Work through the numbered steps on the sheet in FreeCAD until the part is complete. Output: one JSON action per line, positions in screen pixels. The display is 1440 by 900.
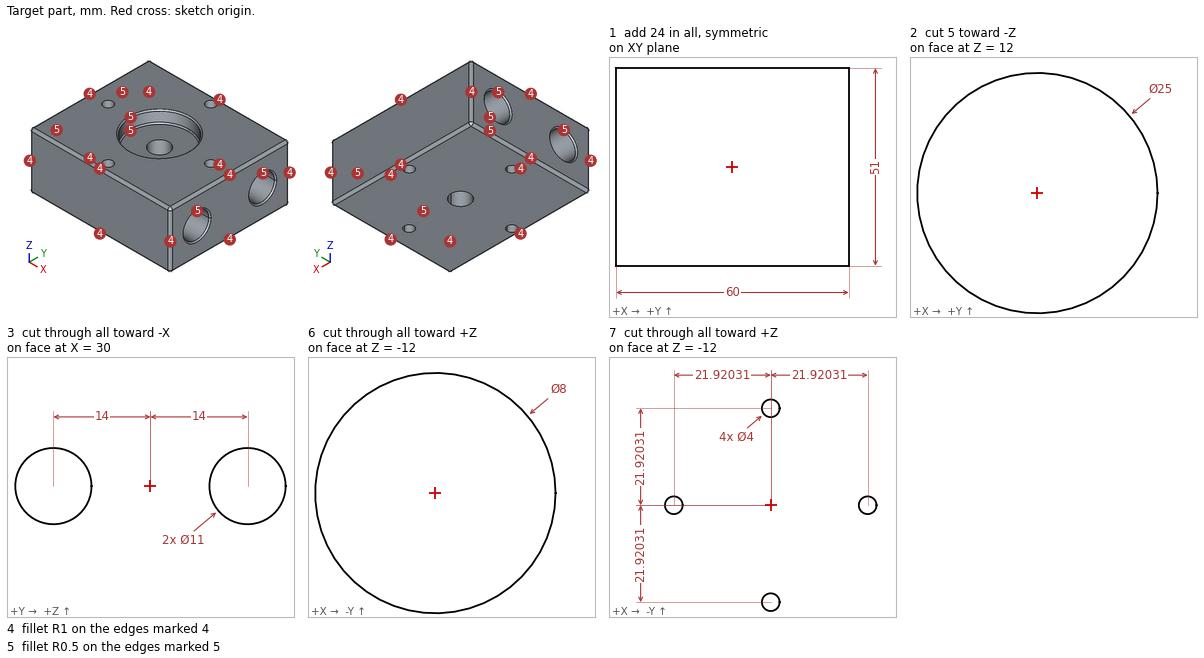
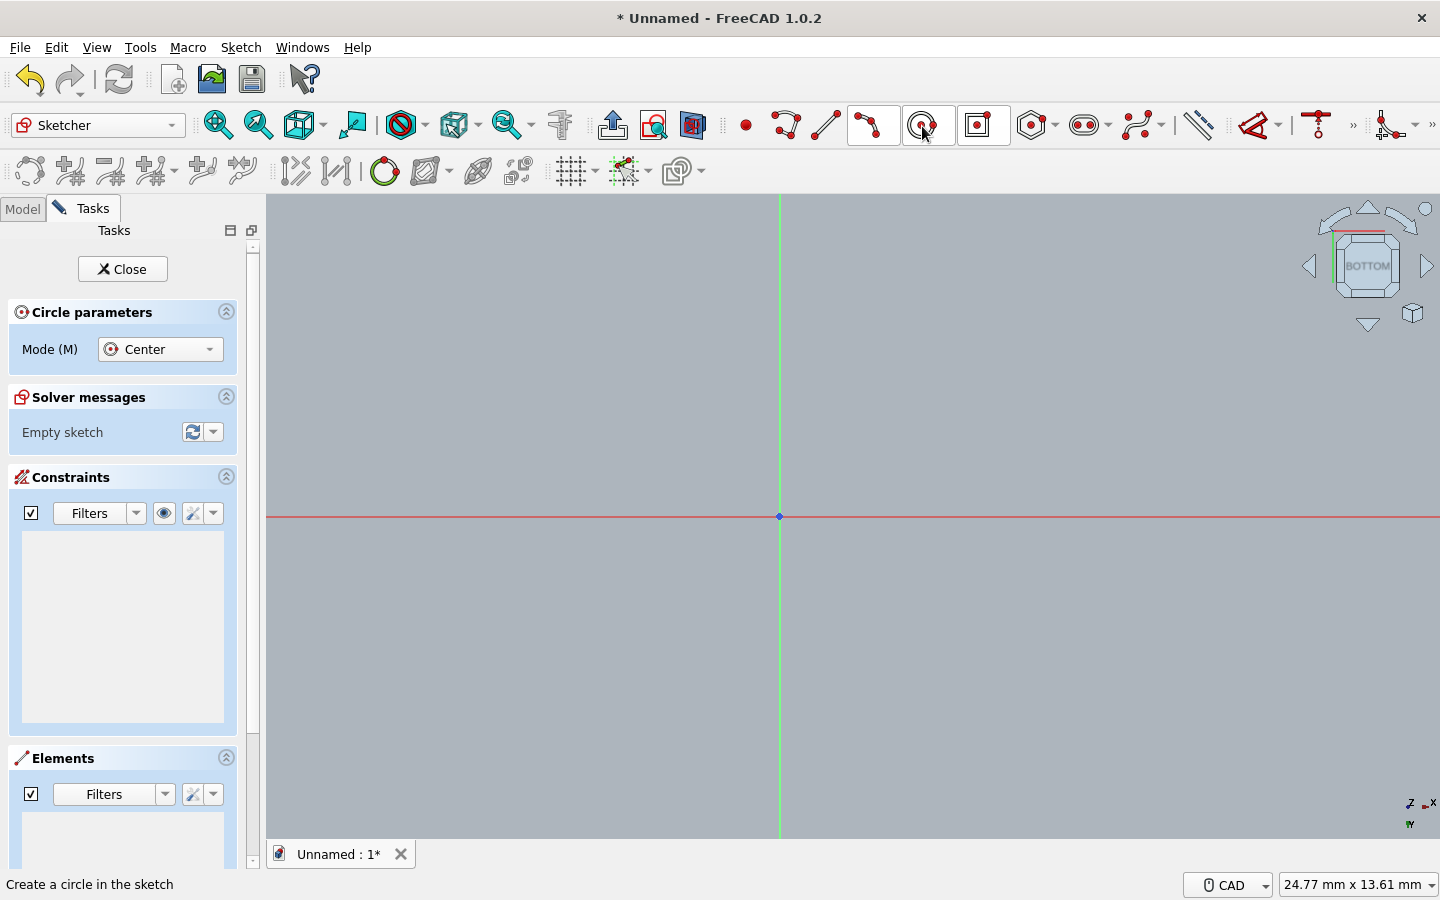
{"action": "left_click", "coordinate": [780, 516]}
{"action": "left_click", "coordinate": [914, 382]}
{"action": "key", "text": "Escape"}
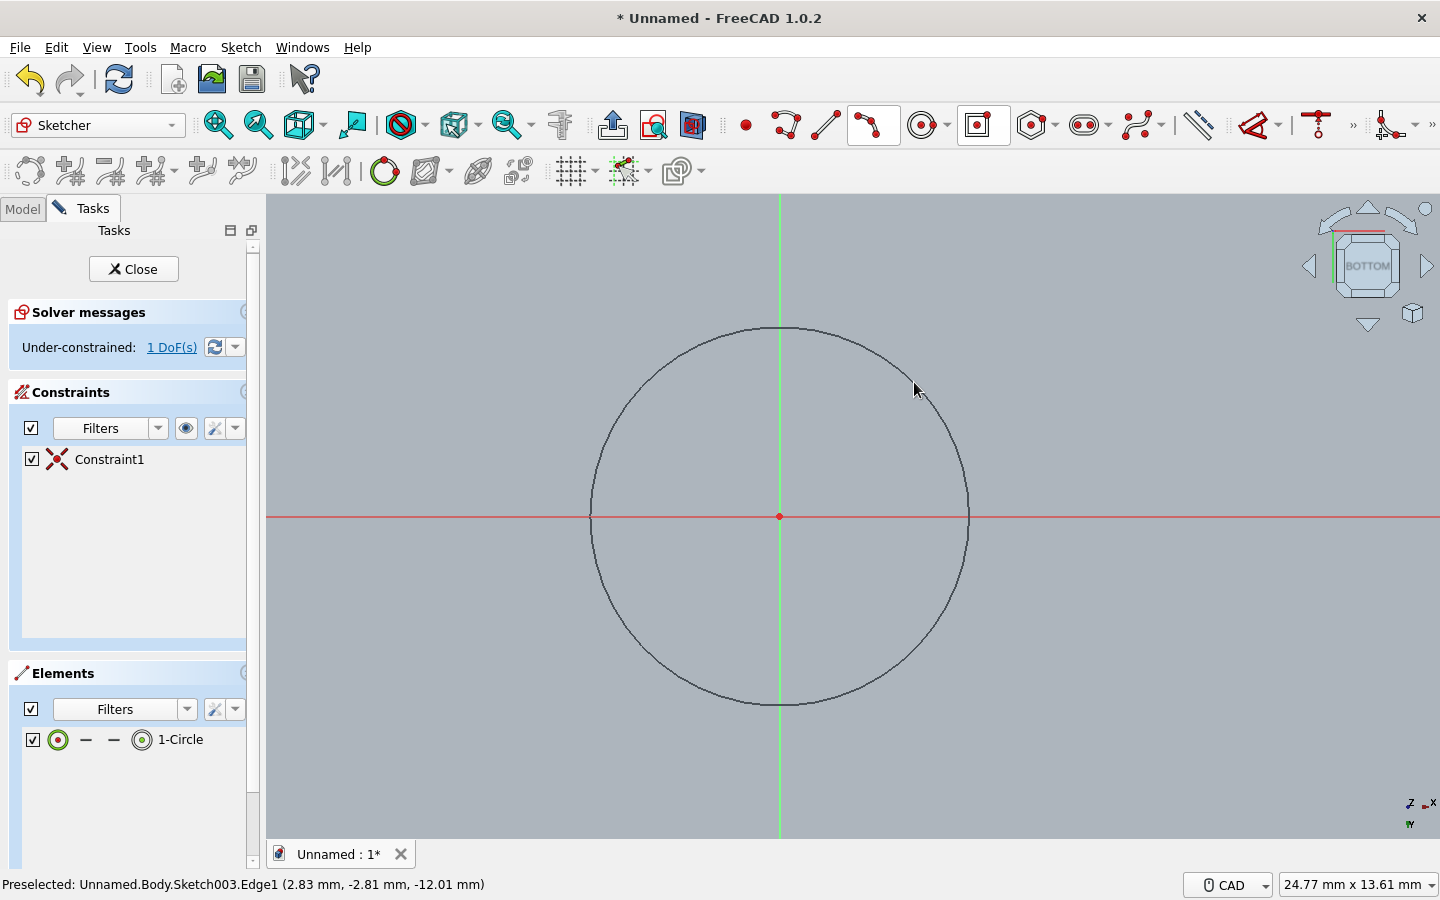
{"action": "left_click", "coordinate": [1254, 126]}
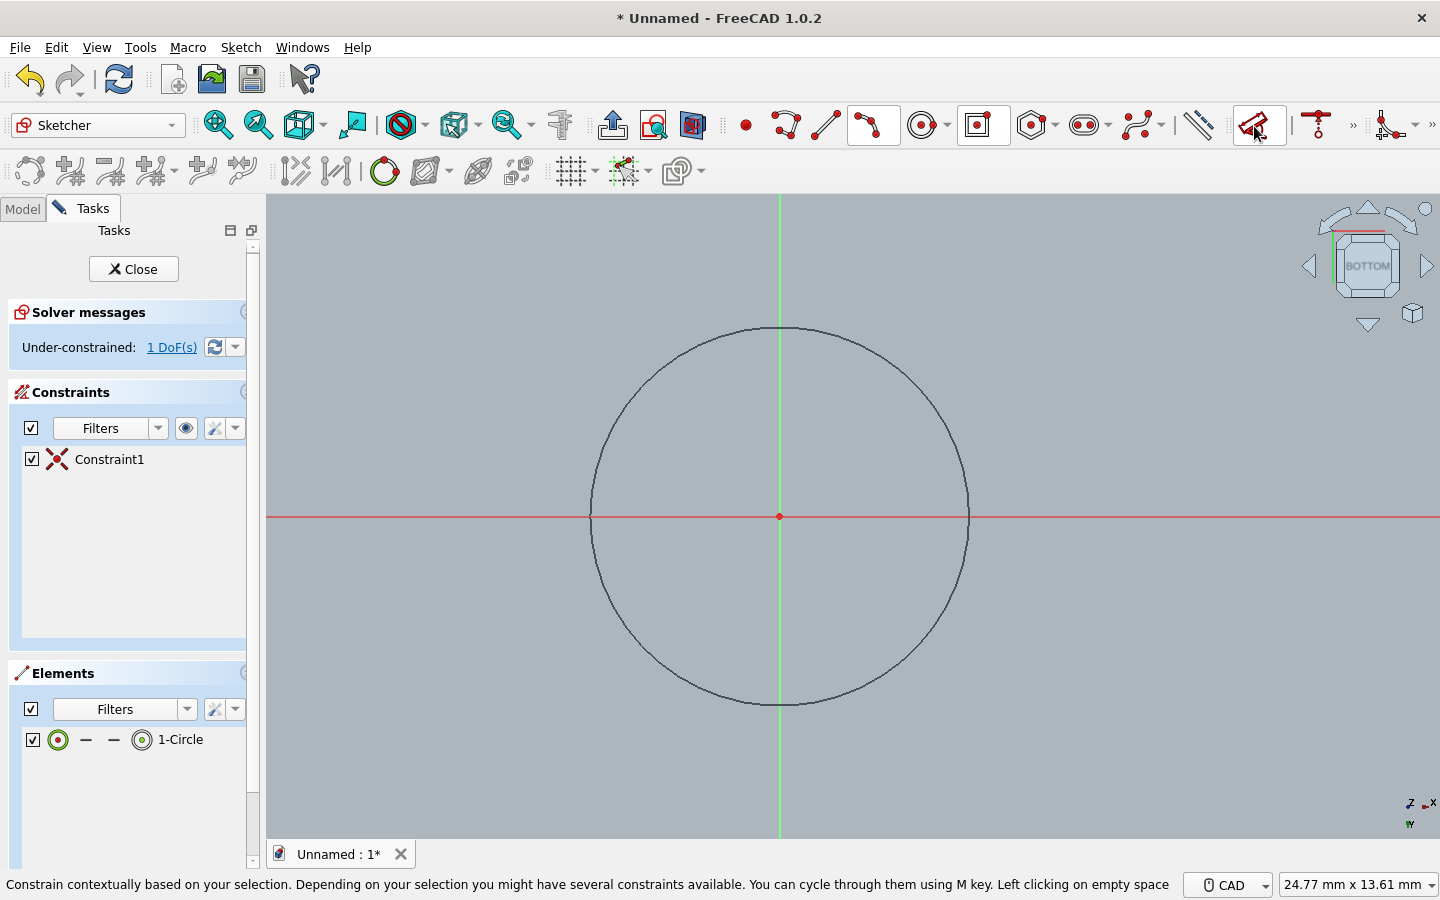
{"action": "left_click", "coordinate": [913, 382]}
{"action": "left_click", "coordinate": [936, 359]}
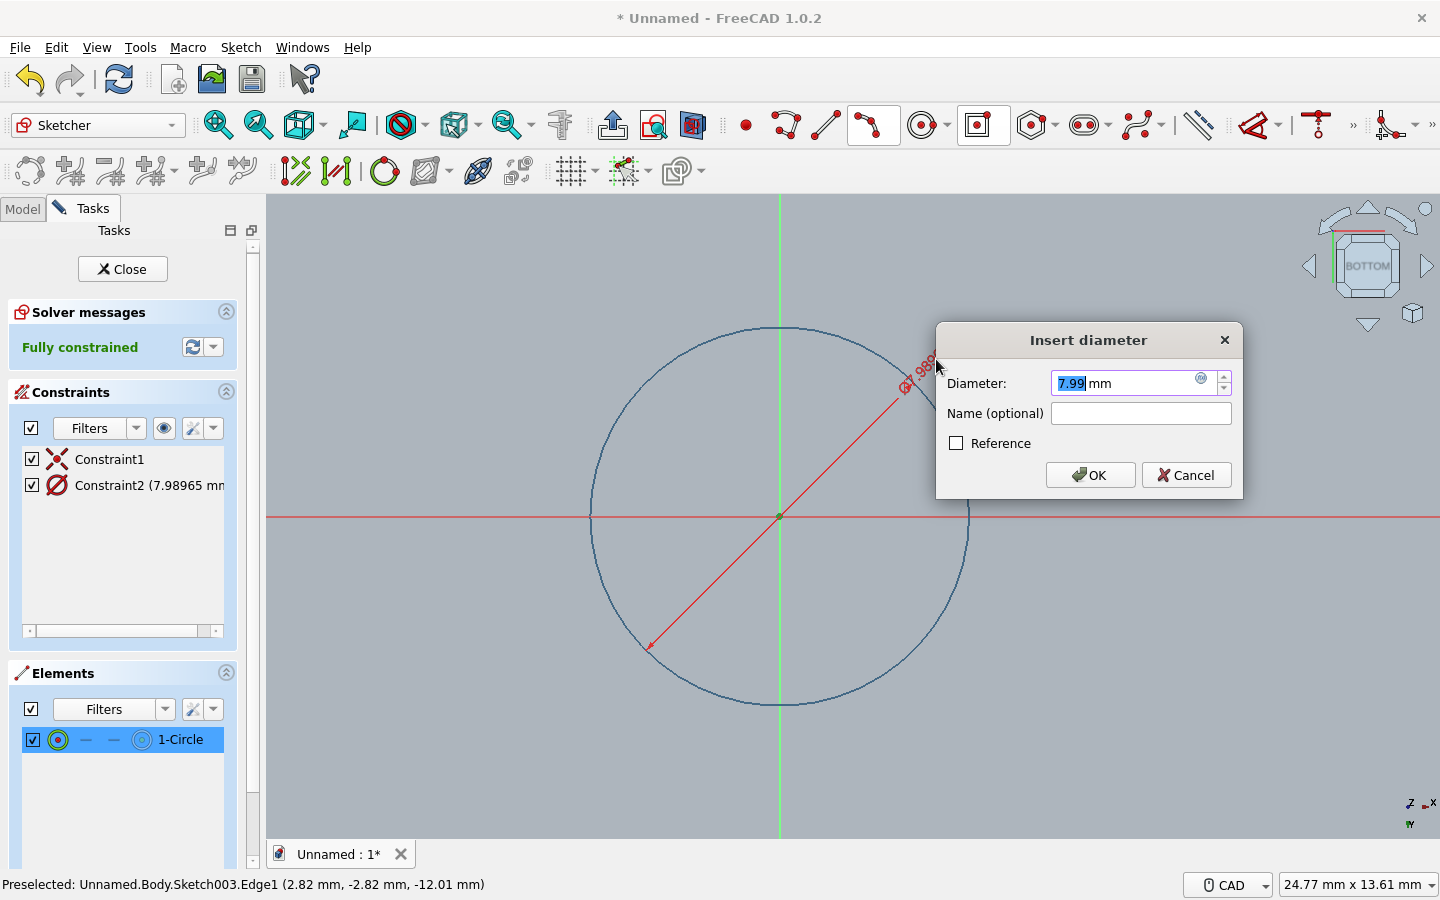
{"action": "type", "text": "8"}
{"action": "key", "text": "Return"}
{"action": "key", "text": "Escape"}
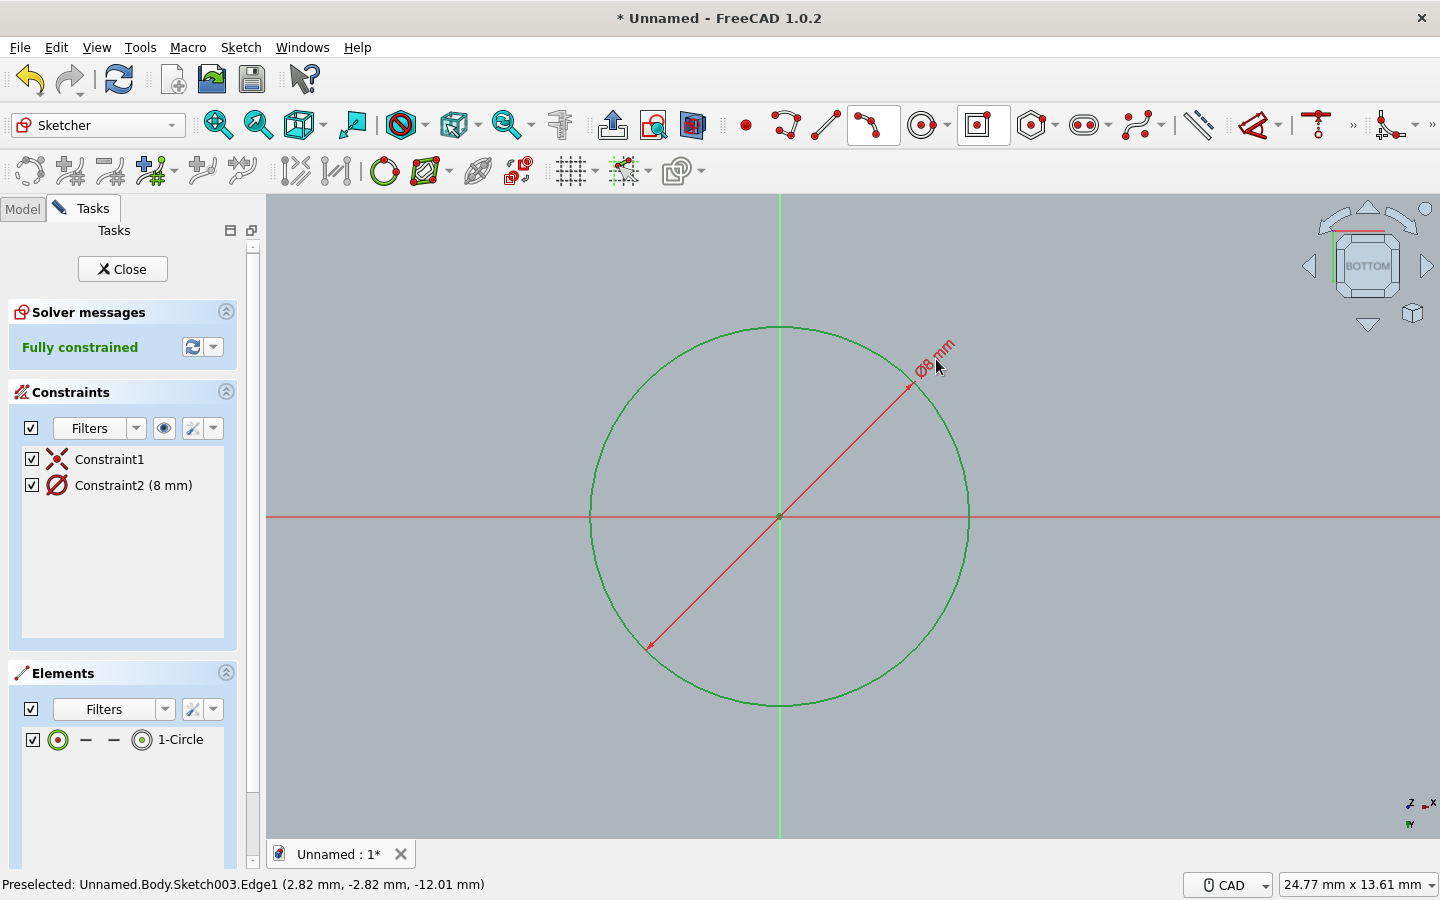
{"action": "left_click", "coordinate": [123, 269]}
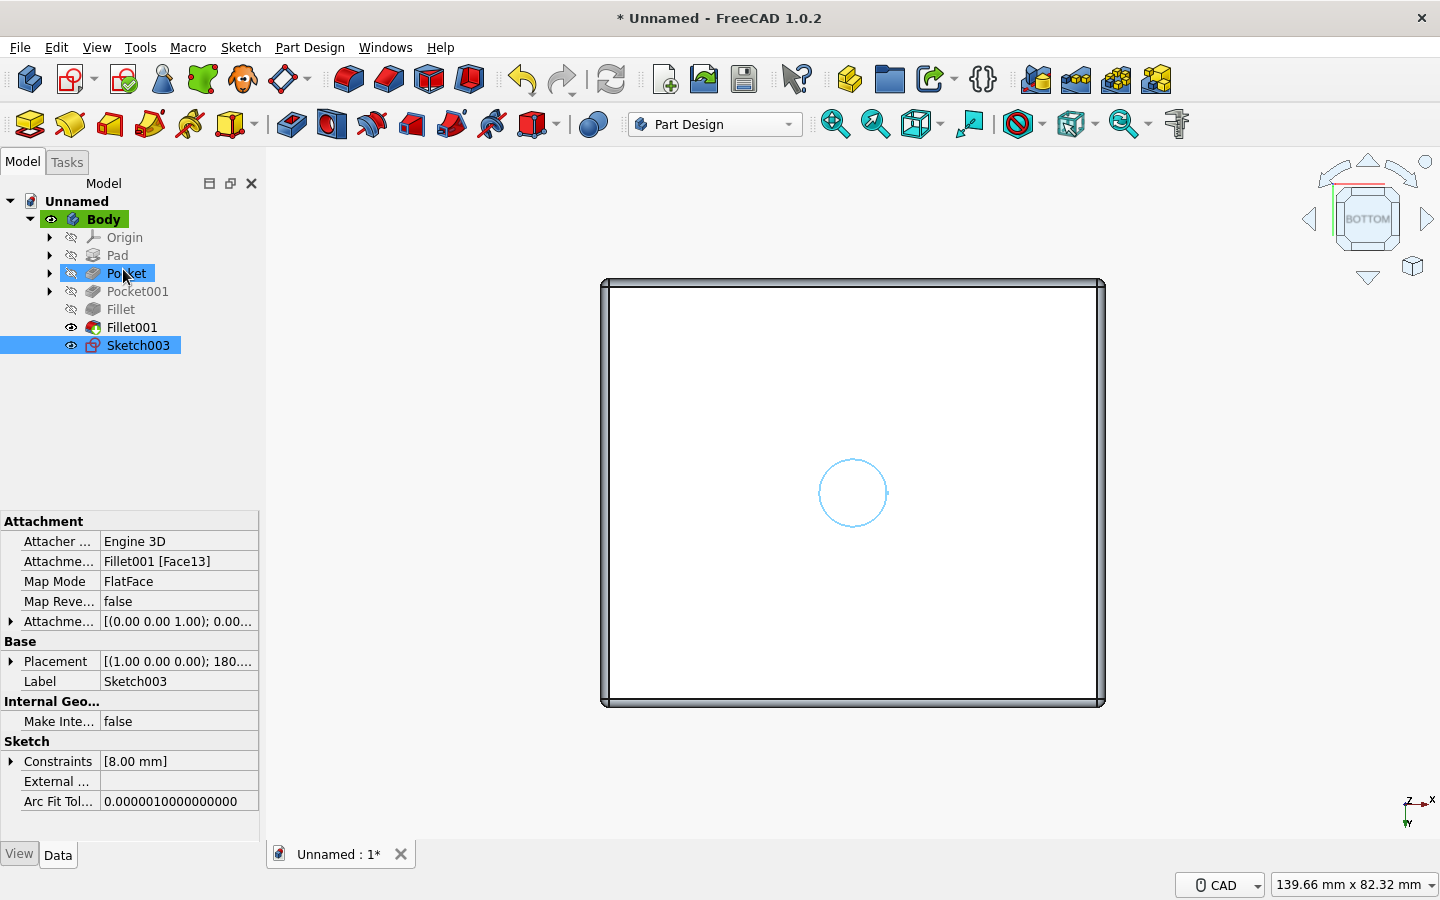
{"action": "left_click", "coordinate": [292, 124]}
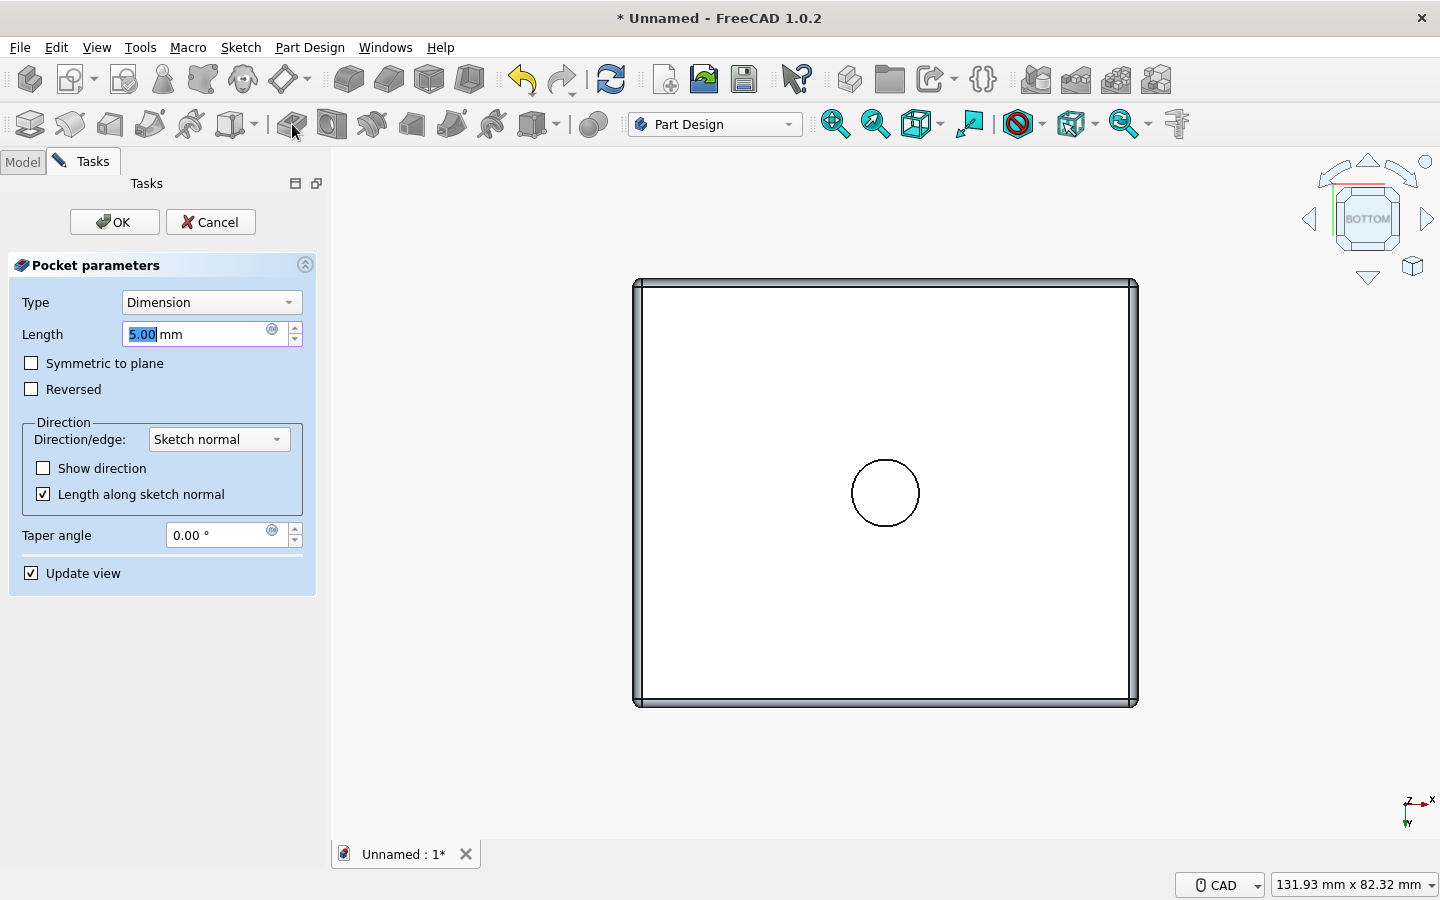
{"action": "left_click", "coordinate": [212, 302]}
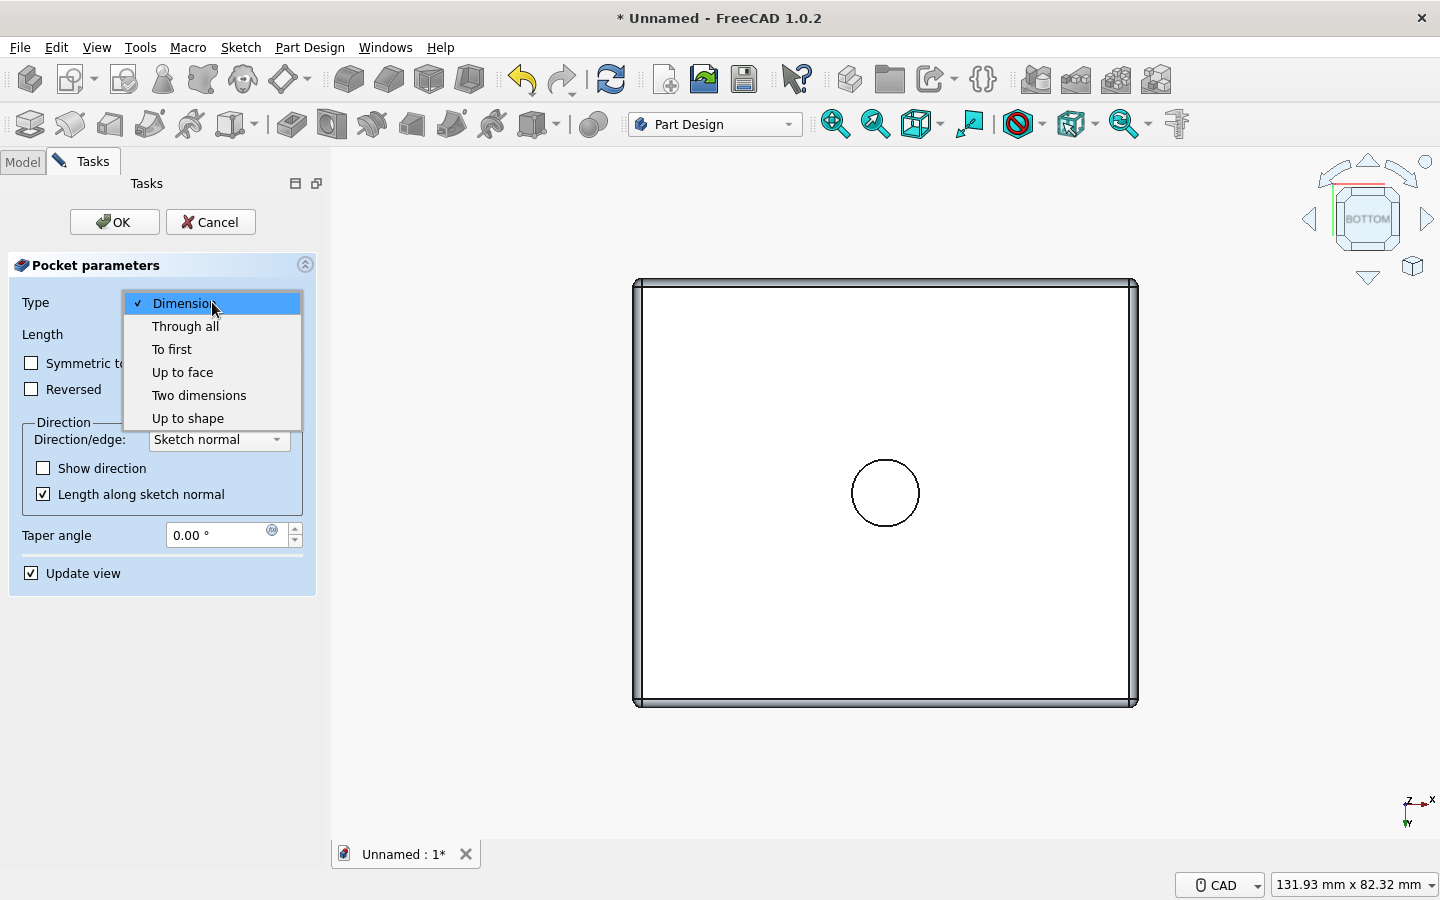
{"action": "left_click", "coordinate": [212, 326]}